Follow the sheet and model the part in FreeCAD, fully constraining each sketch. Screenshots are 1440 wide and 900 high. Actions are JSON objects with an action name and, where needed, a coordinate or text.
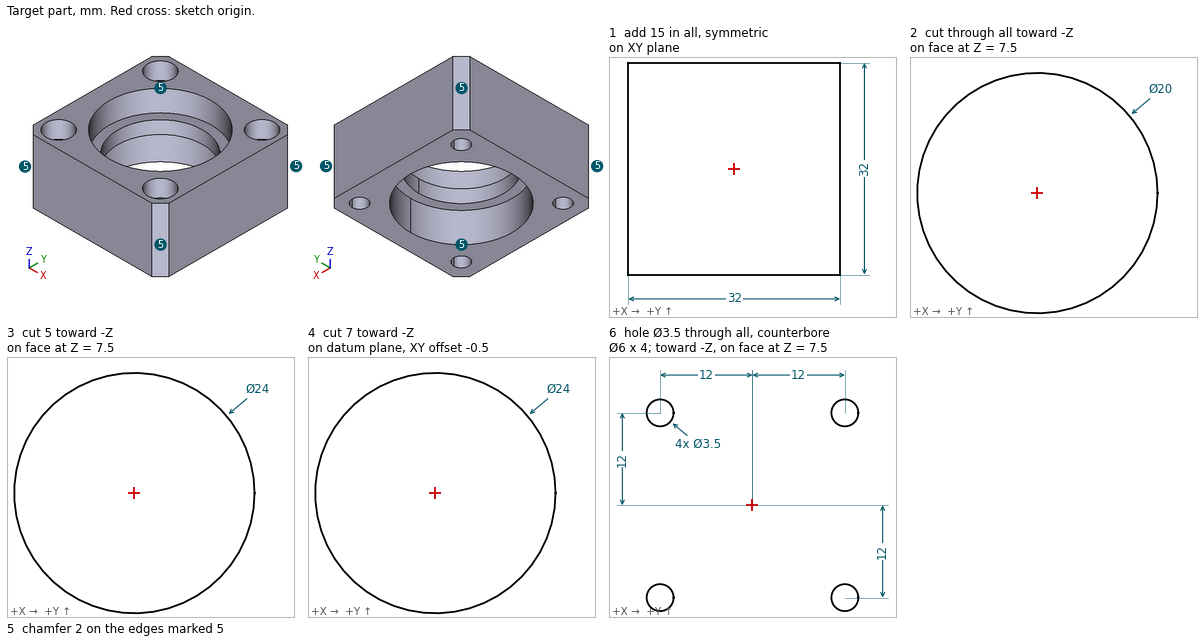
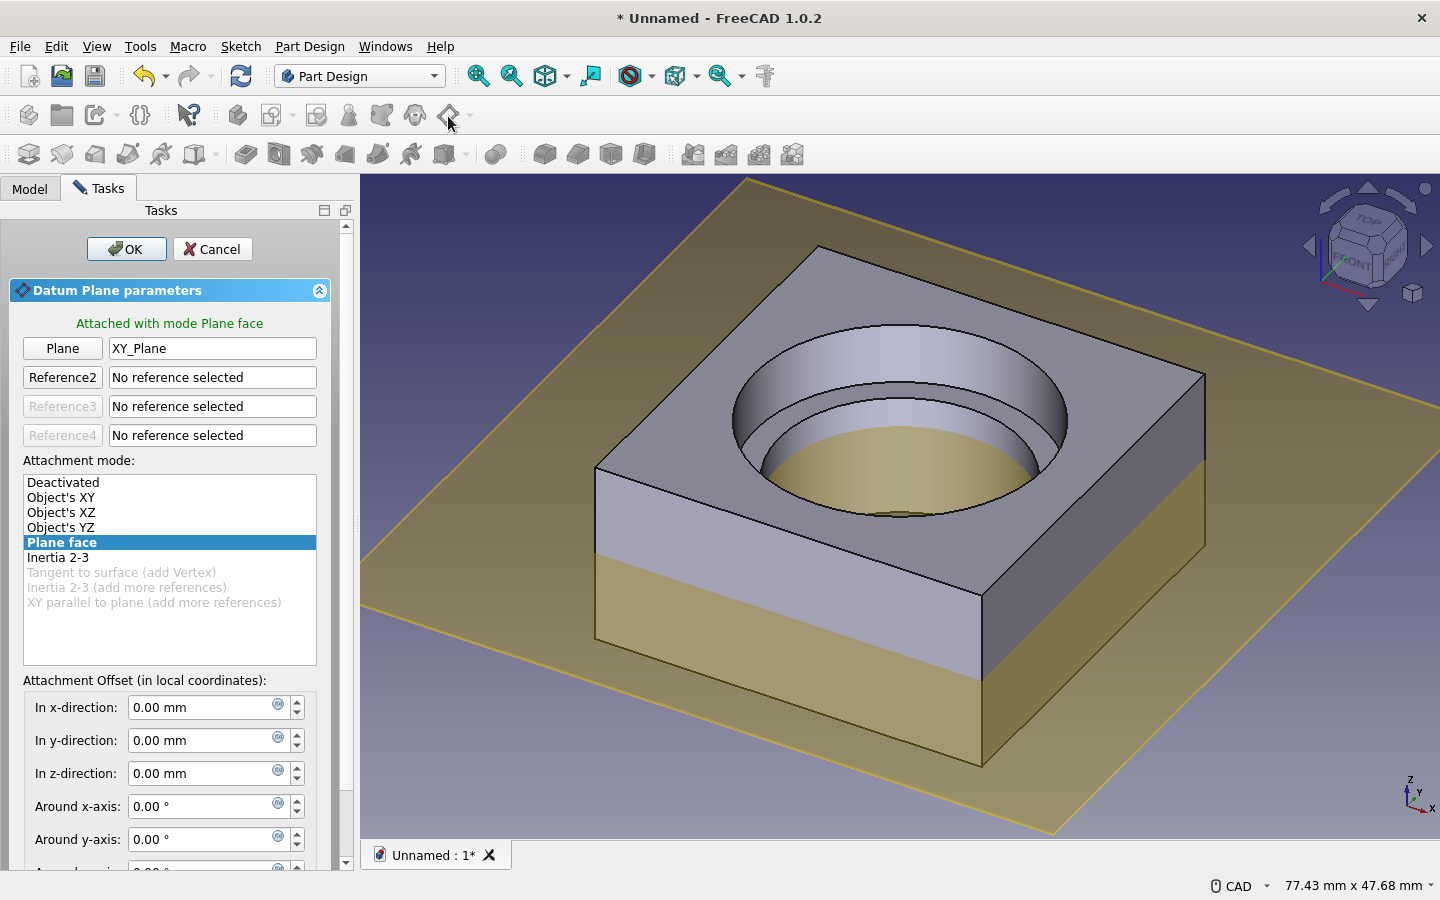
{"action": "triple_click", "coordinate": [210, 774]}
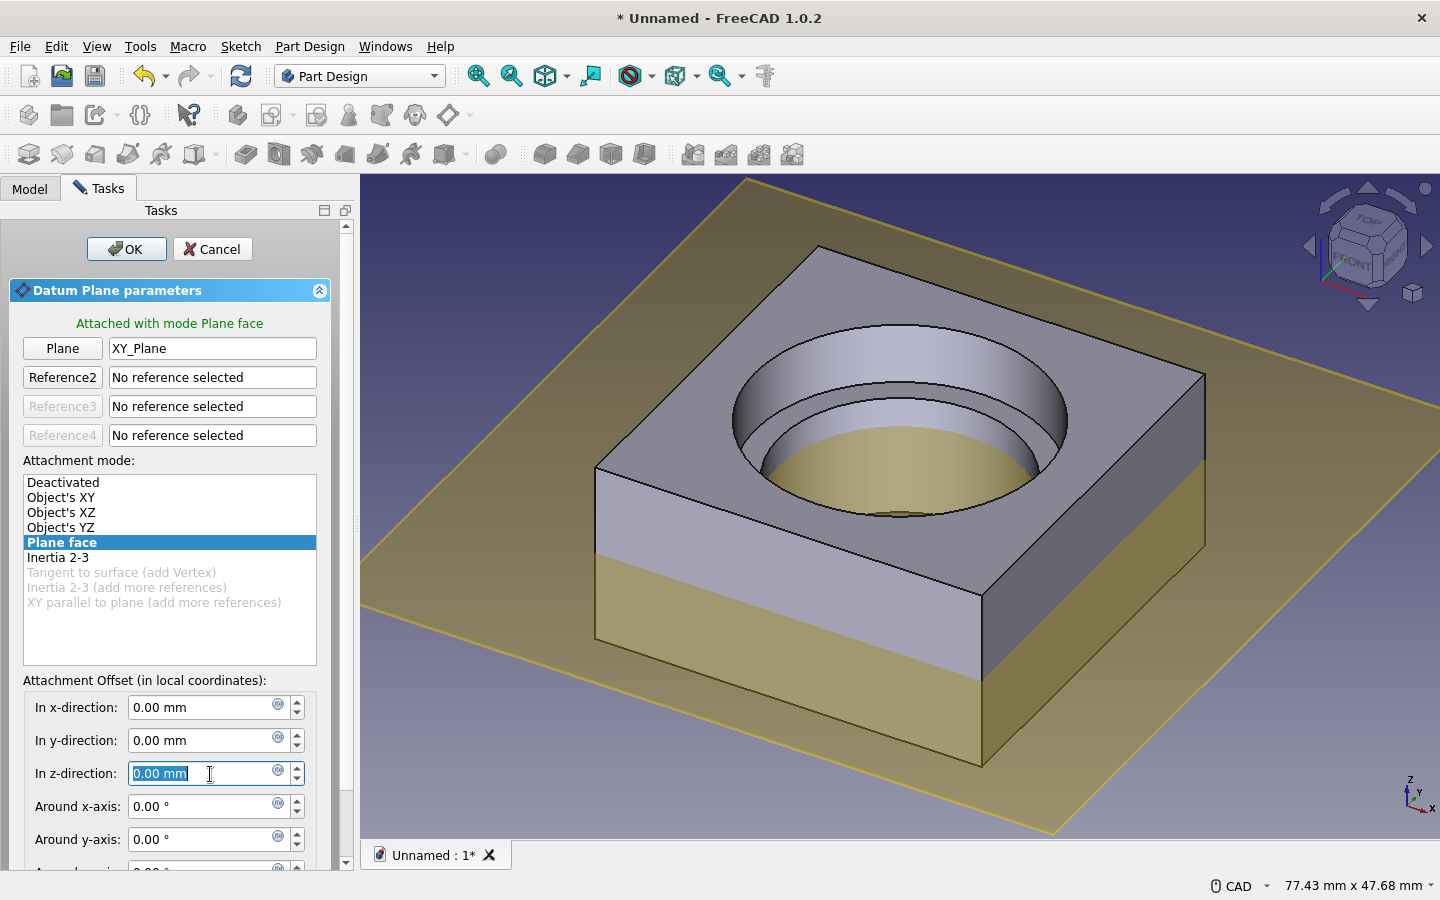
{"action": "type", "text": "-0.5"}
{"action": "key", "text": "Tab"}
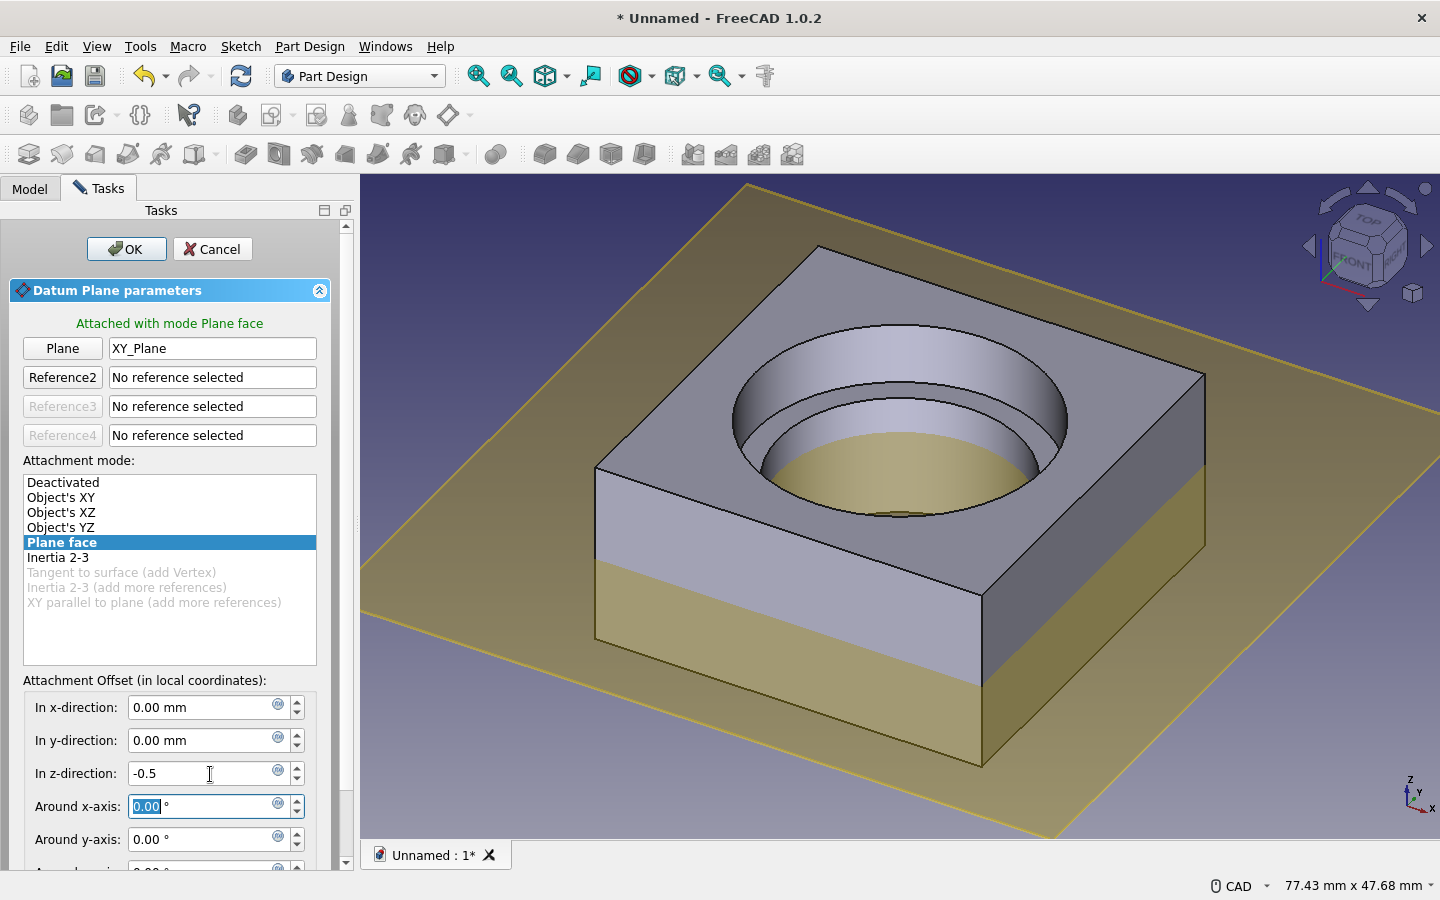
{"action": "left_click", "coordinate": [127, 249]}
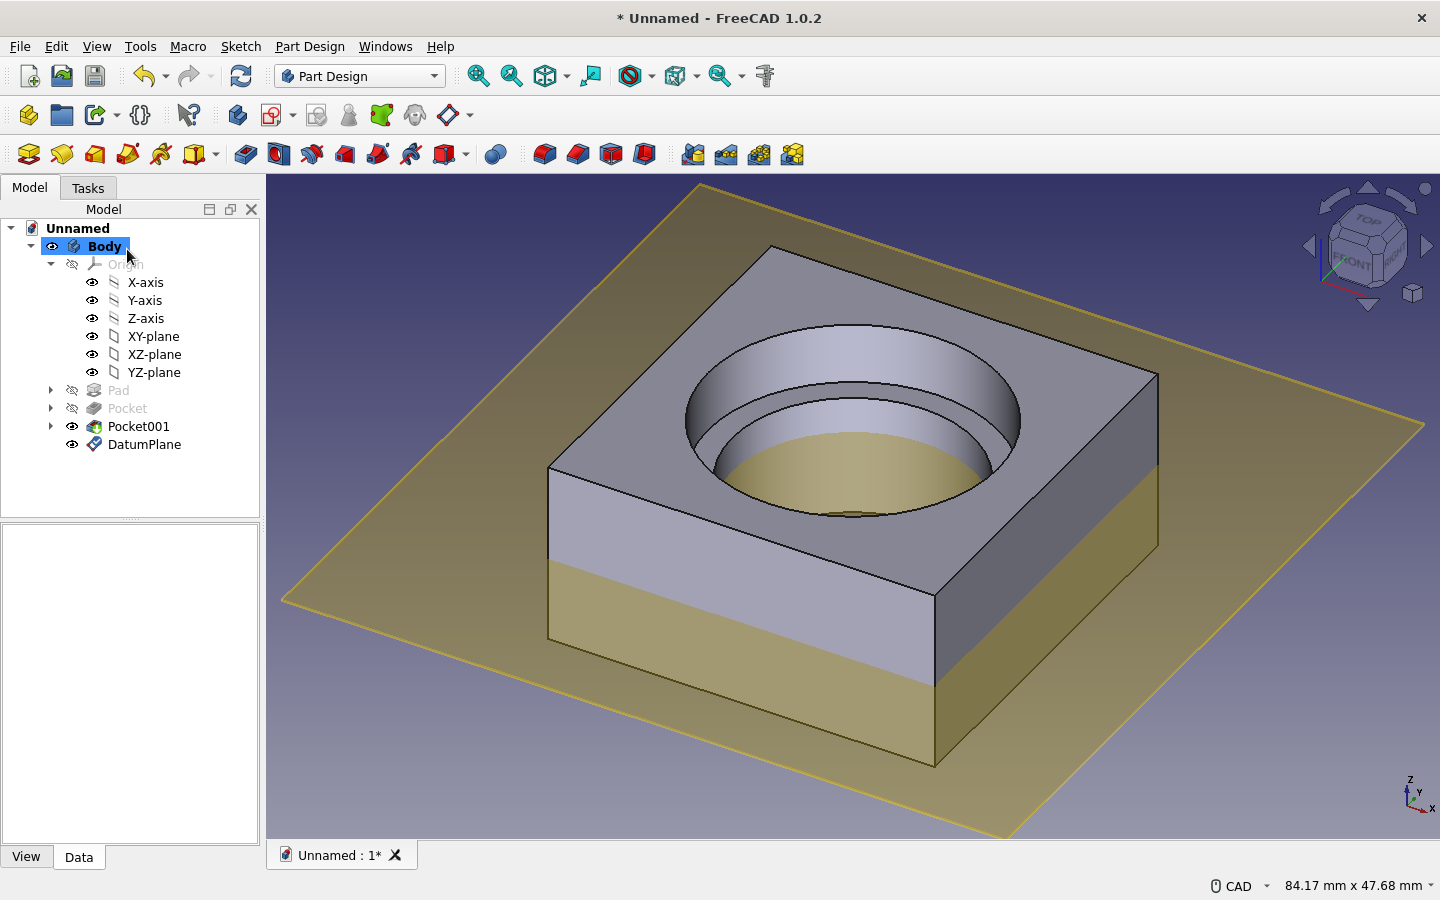
{"action": "left_click", "coordinate": [117, 444]}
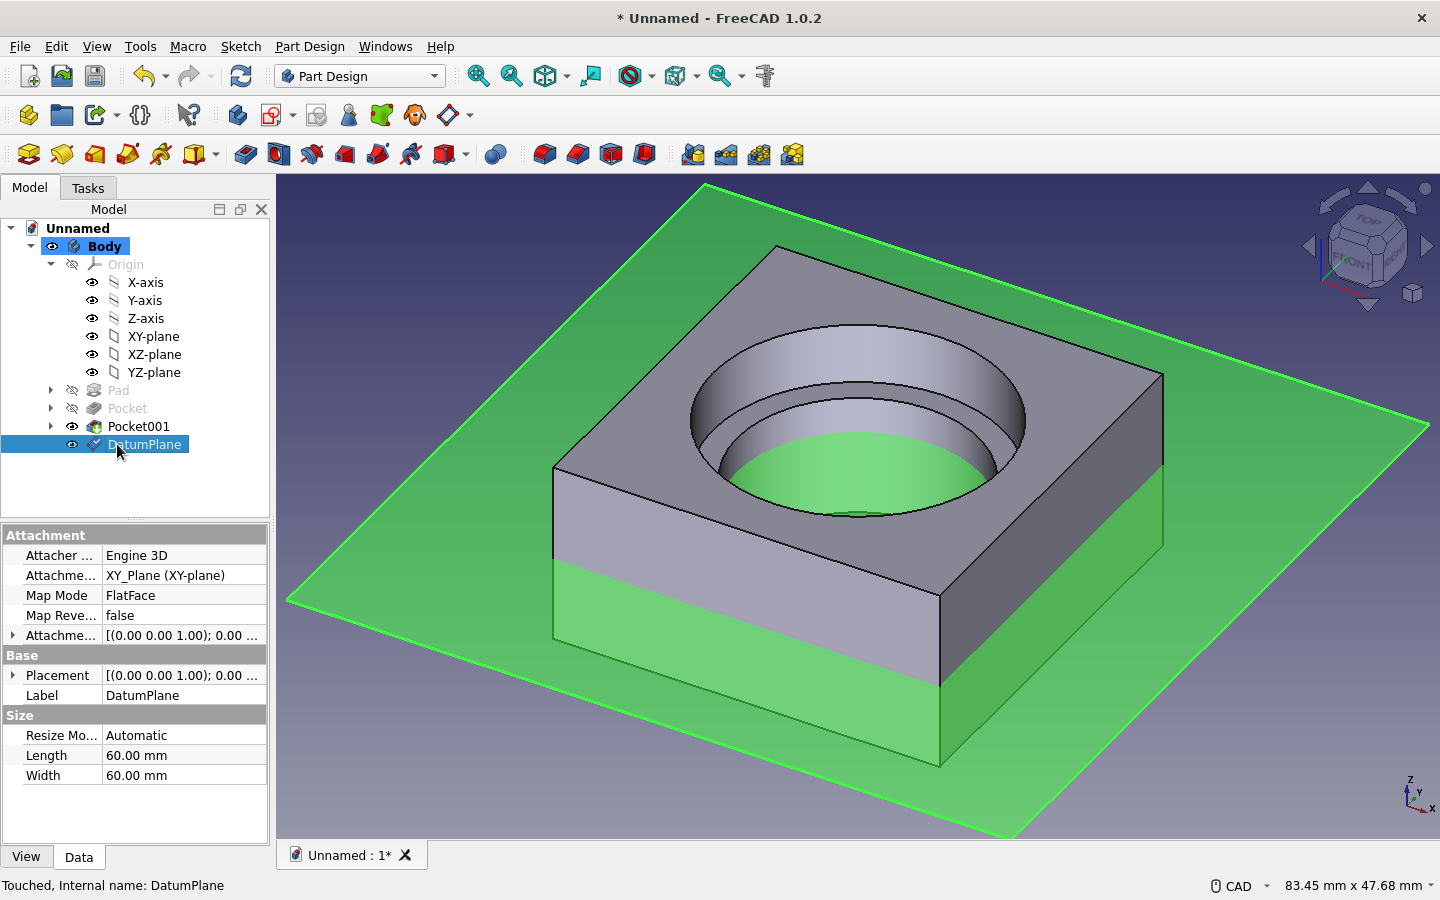
{"action": "left_click", "coordinate": [270, 116]}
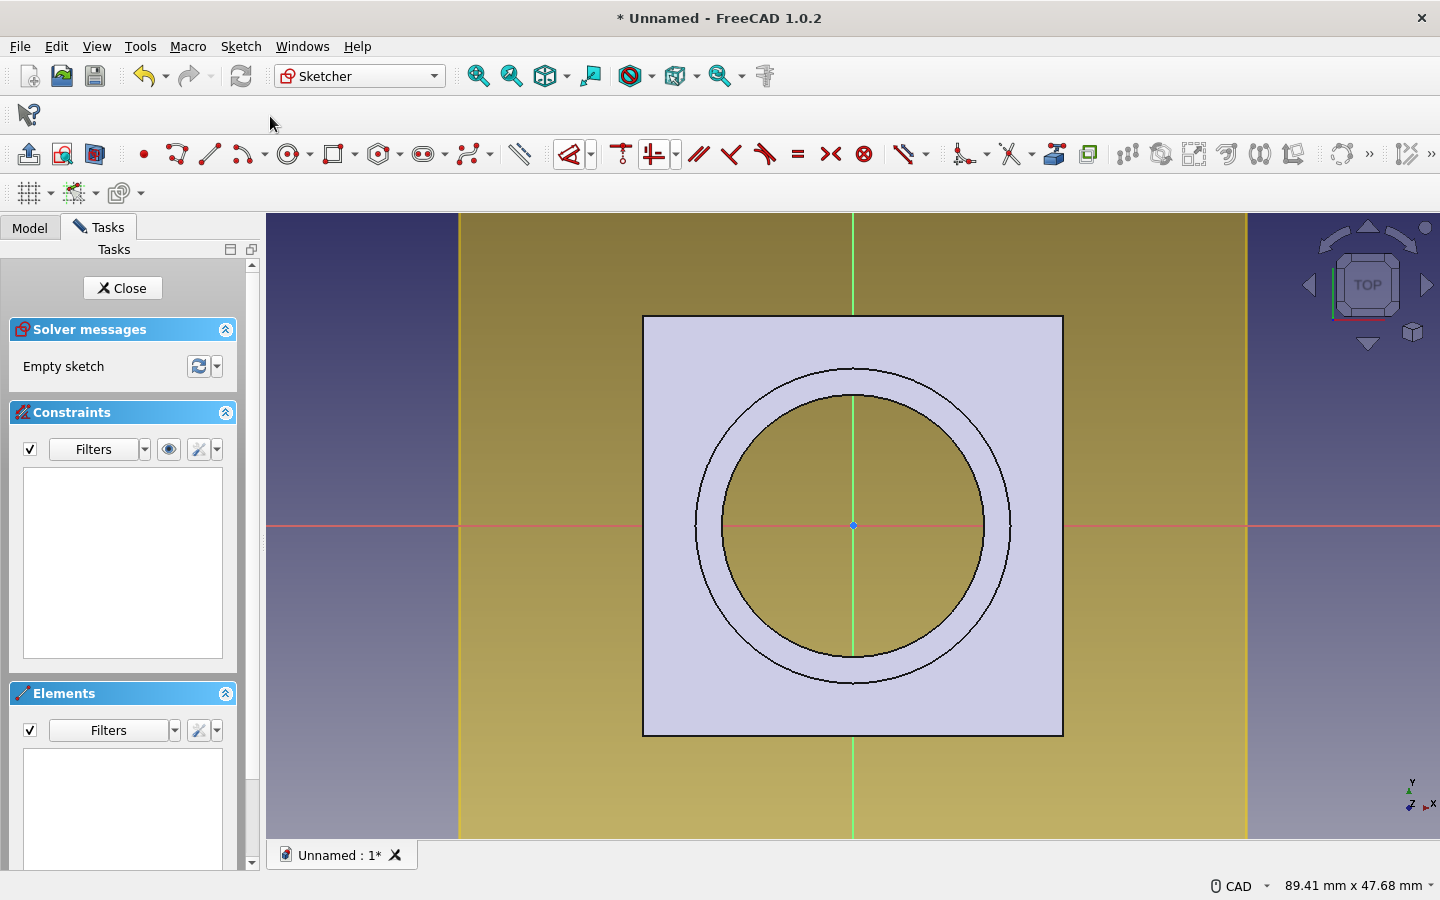
{"action": "left_click", "coordinate": [95, 154]}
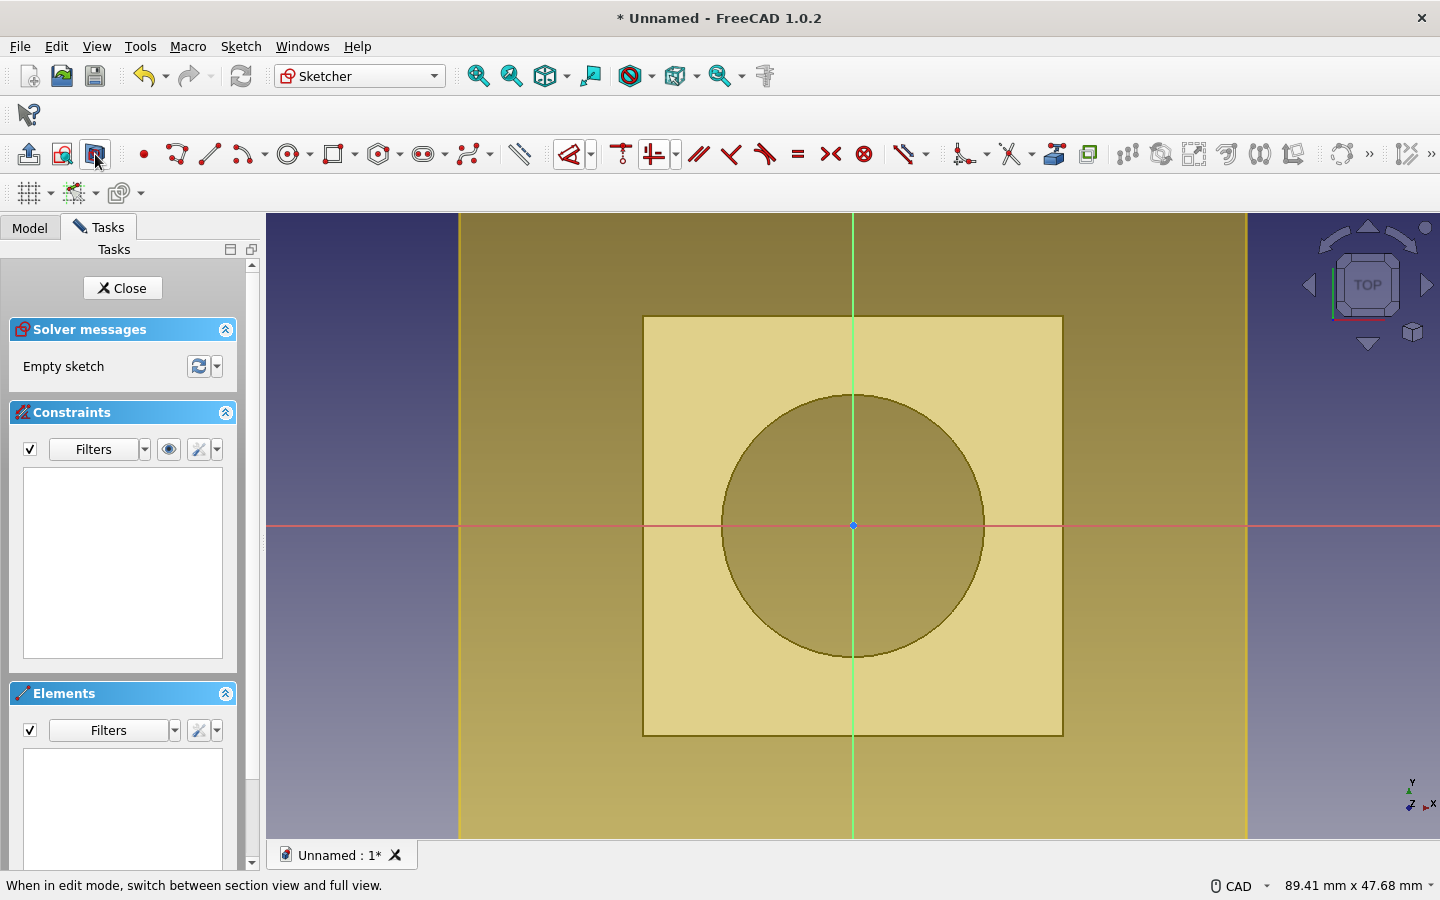
{"action": "left_click", "coordinate": [288, 154]}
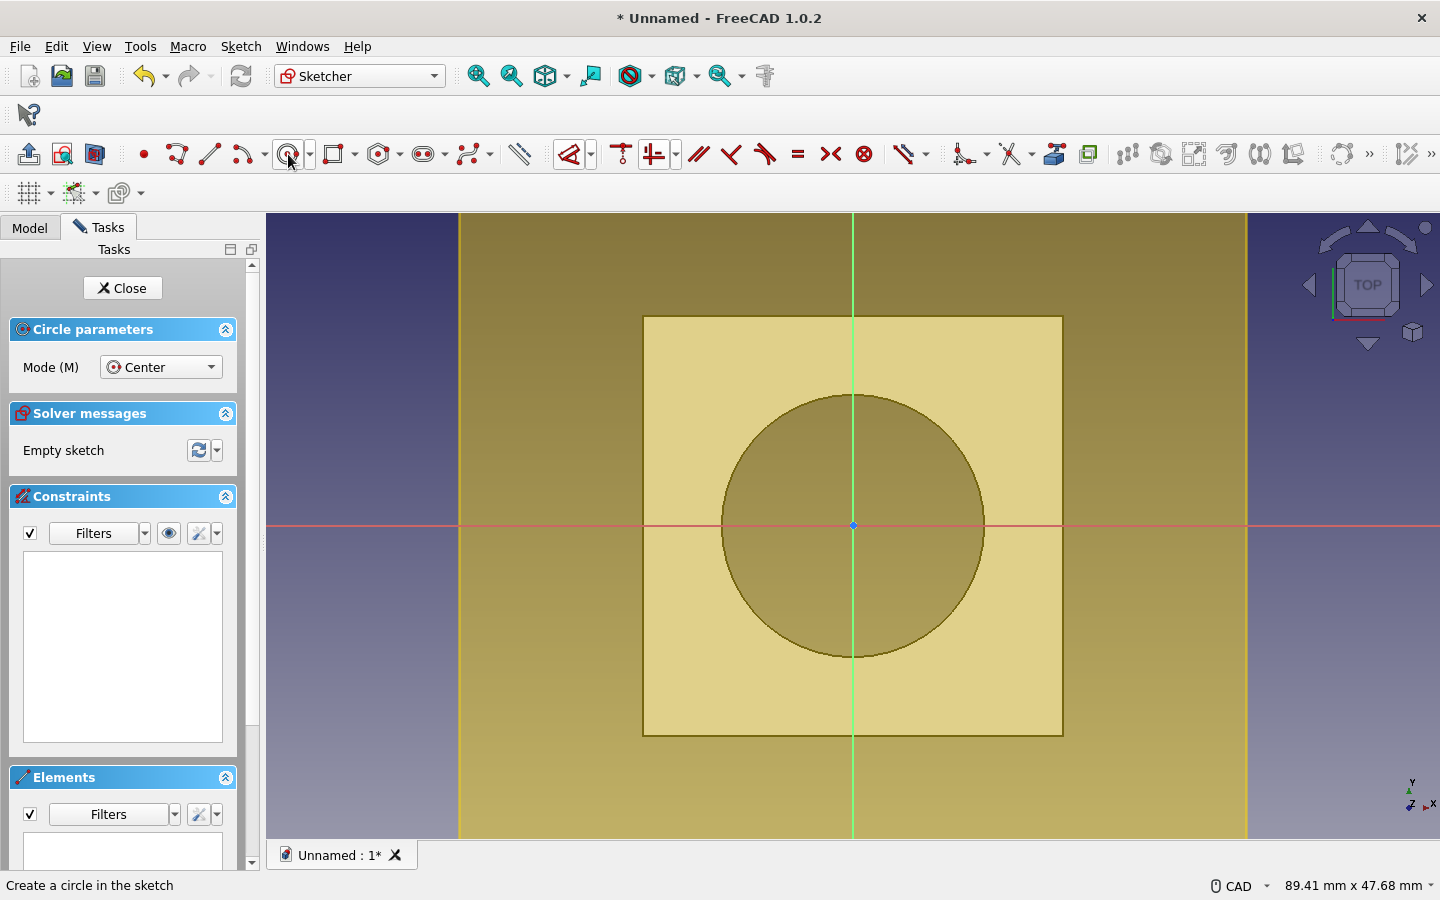
{"action": "left_click", "coordinate": [853, 526]}
{"action": "left_click", "coordinate": [964, 415]}
{"action": "key", "text": "Escape"}